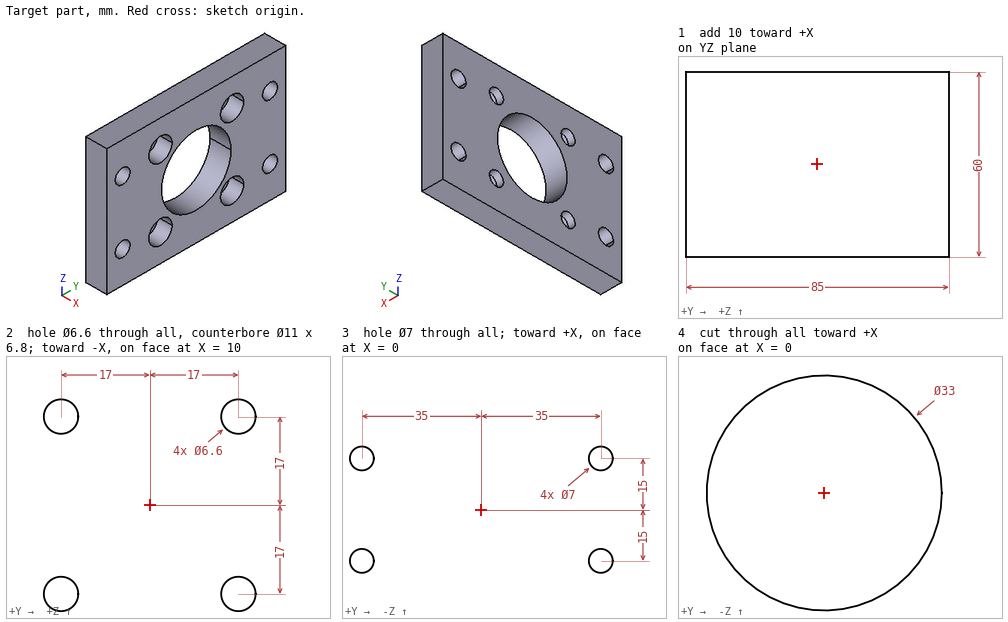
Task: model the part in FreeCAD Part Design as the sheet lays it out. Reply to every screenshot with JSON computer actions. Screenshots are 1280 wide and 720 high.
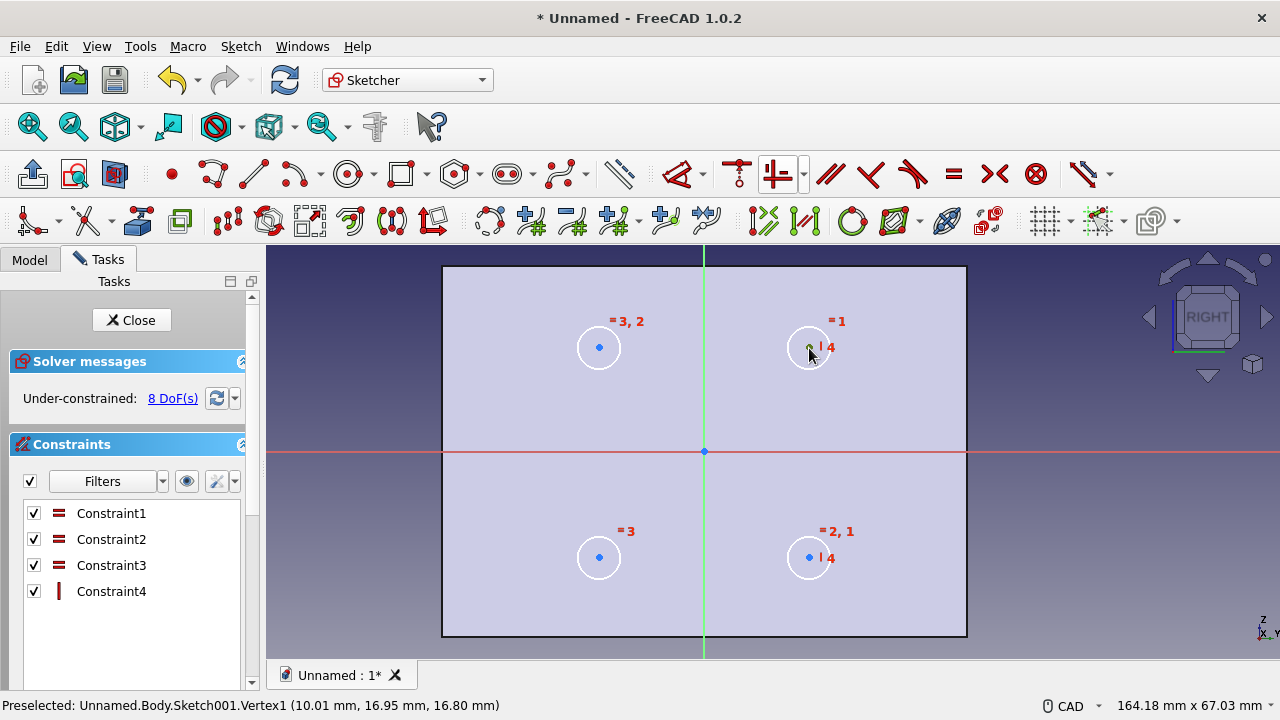
{"action": "left_click", "coordinate": [599, 348]}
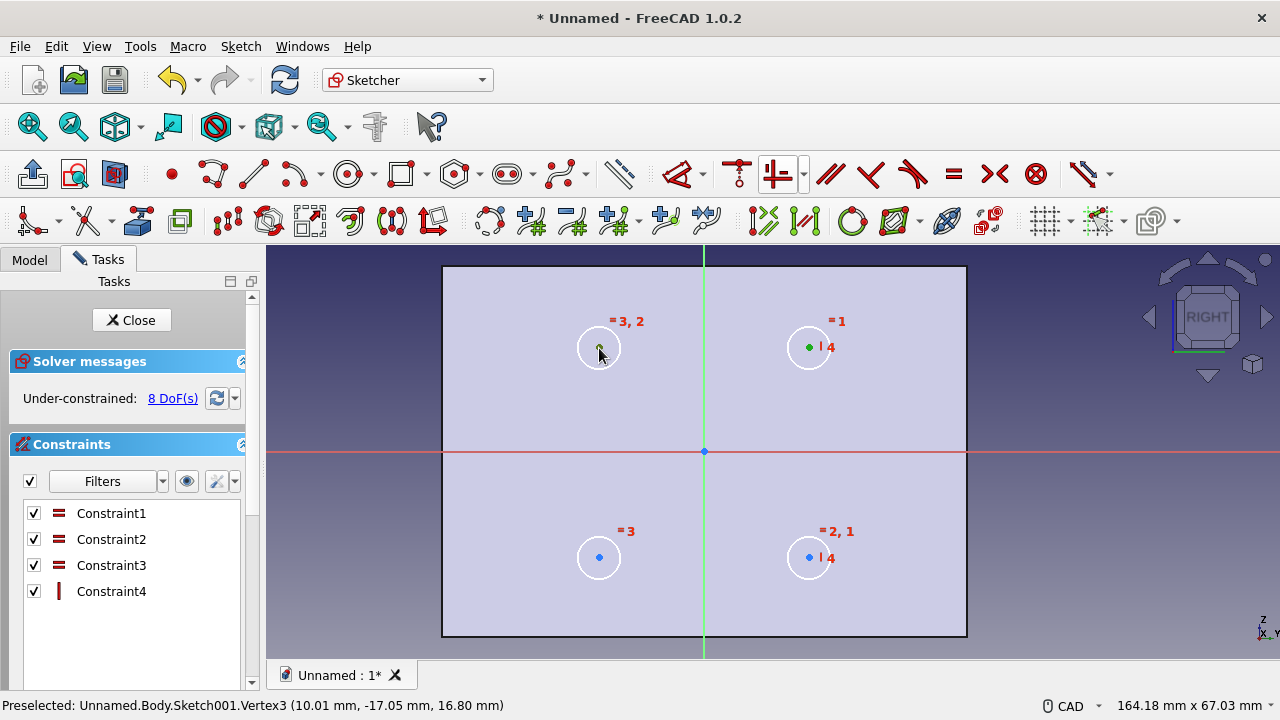
{"action": "key", "text": "h"}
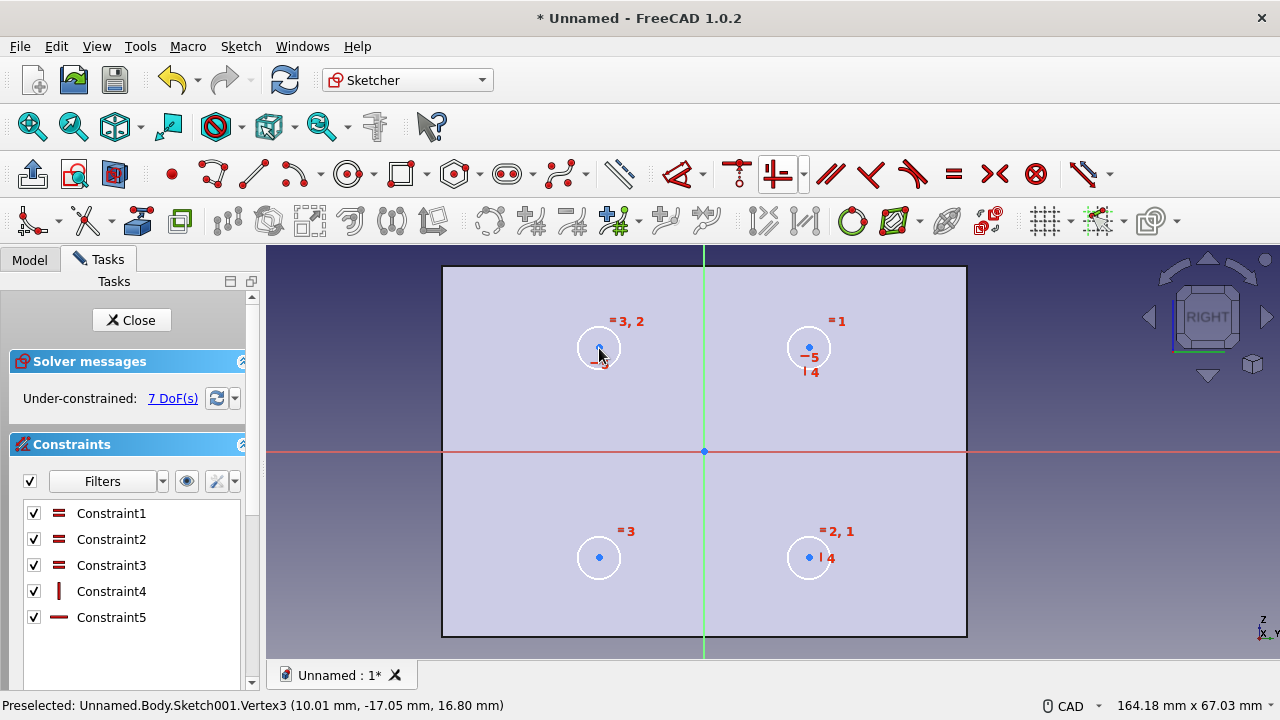
{"action": "left_click", "coordinate": [599, 348]}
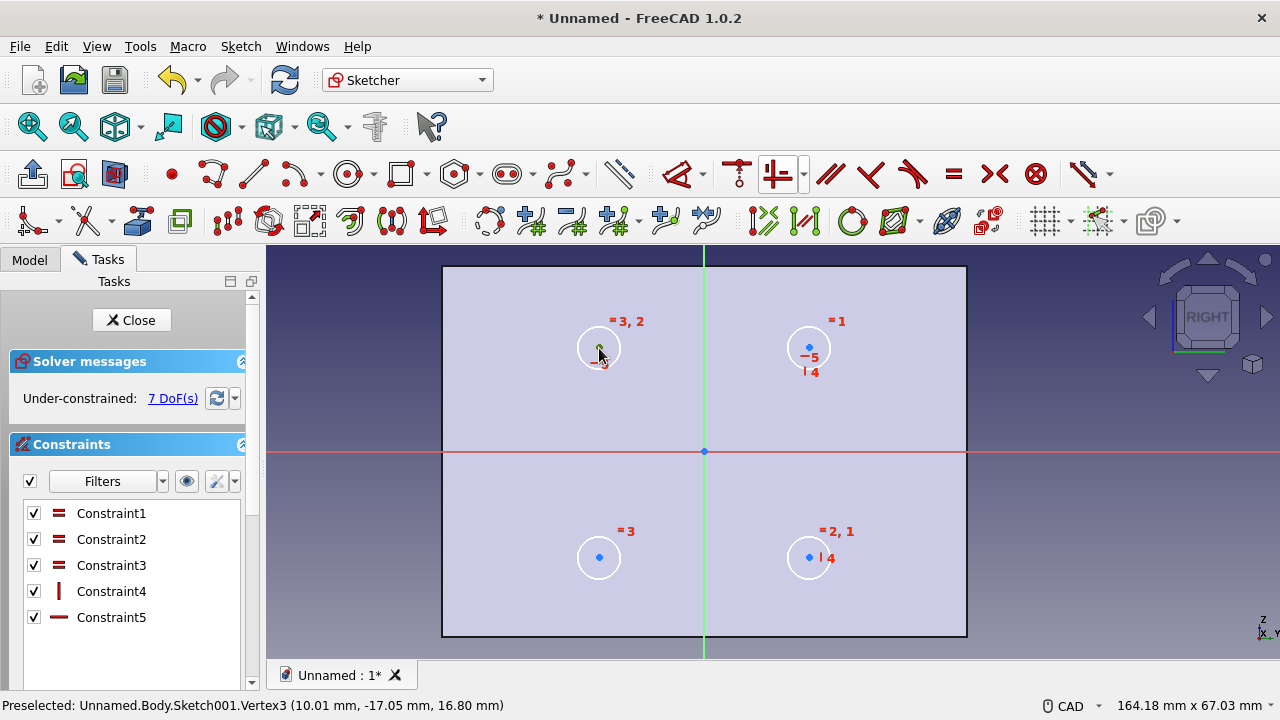
{"action": "left_click", "coordinate": [599, 558]}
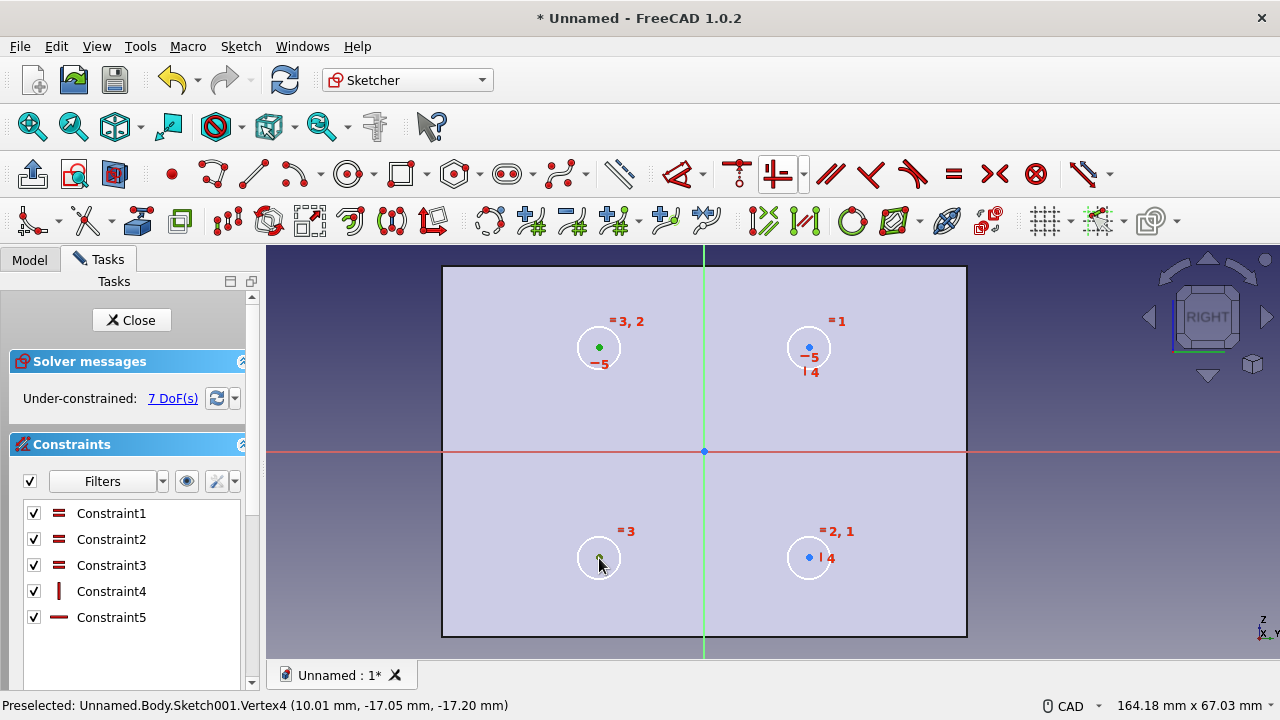
{"action": "key", "text": "v"}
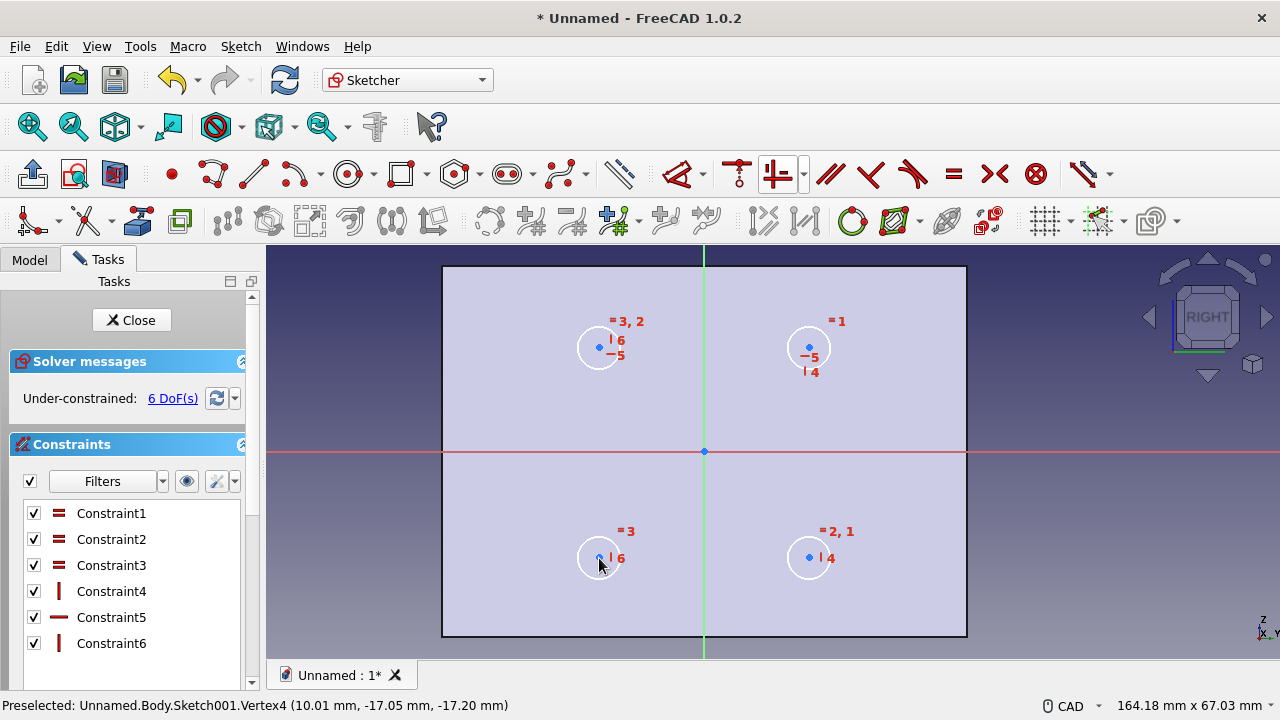
{"action": "left_click", "coordinate": [809, 558]}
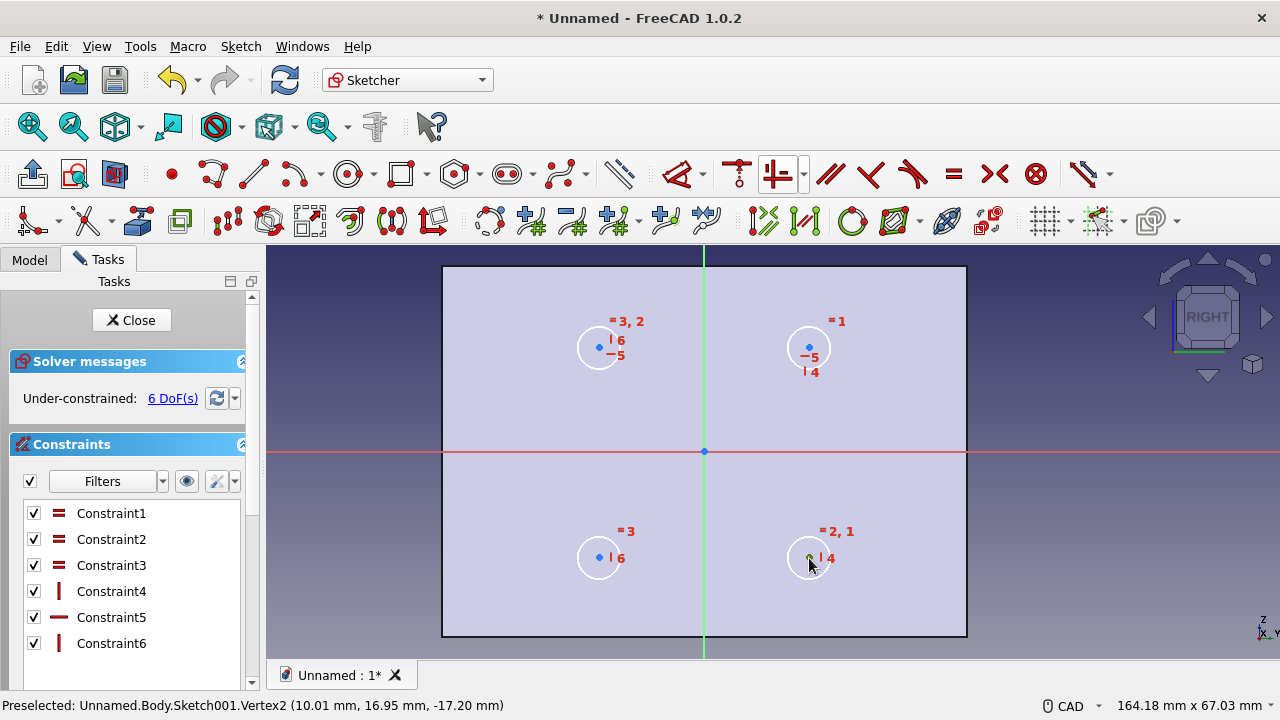
{"action": "left_click", "coordinate": [599, 558]}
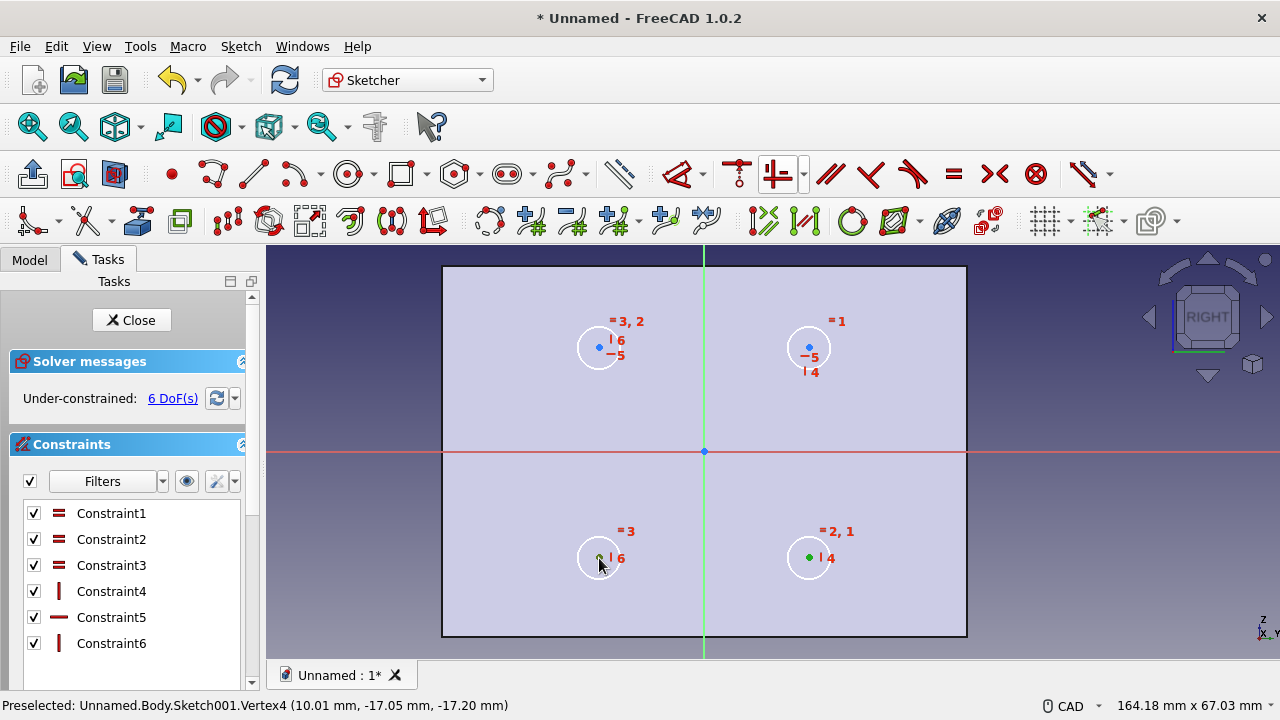
{"action": "key", "text": "h"}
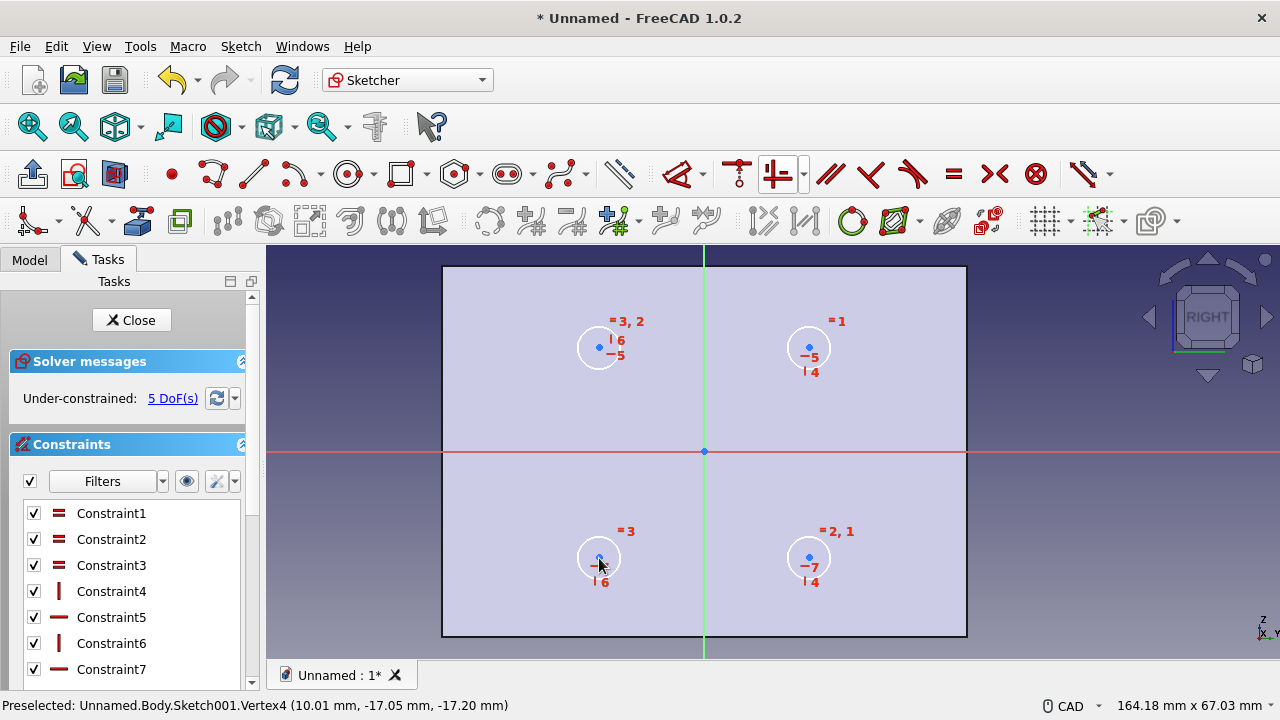
{"action": "left_click", "coordinate": [824, 333]}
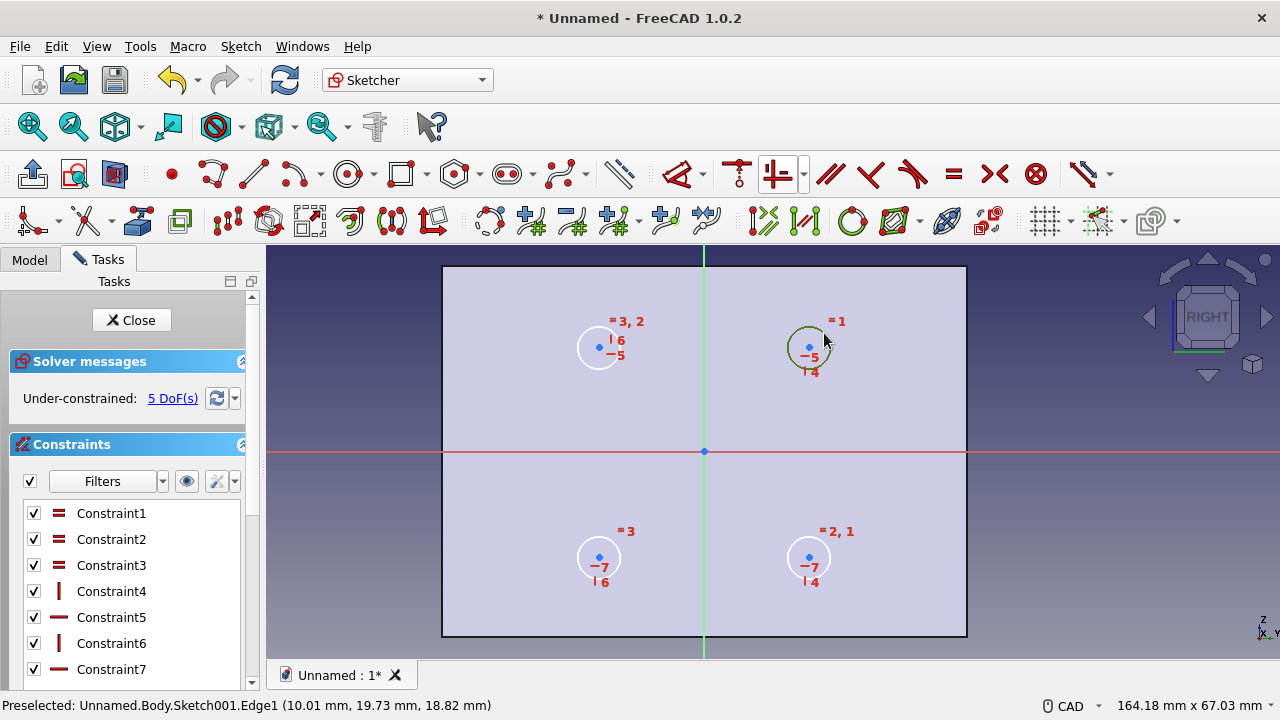
{"action": "key", "text": "k o"}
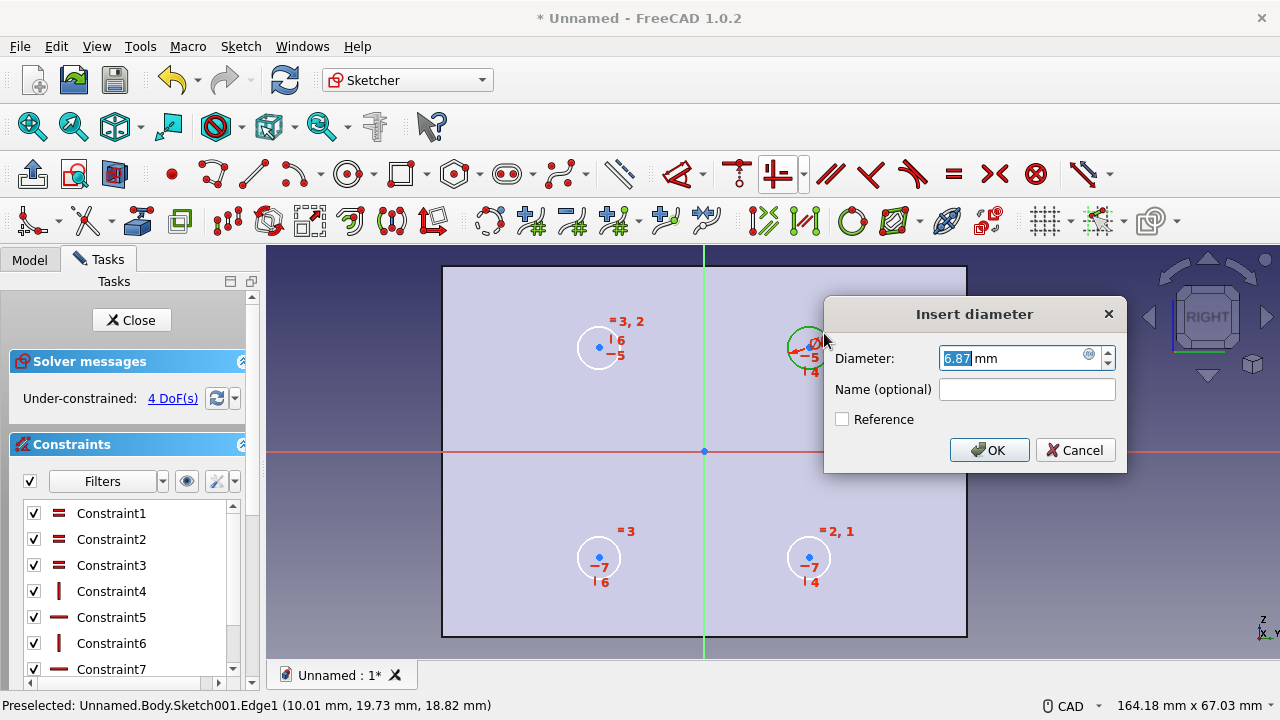
{"action": "type", "text": "6.6"}
{"action": "key", "text": "Return"}